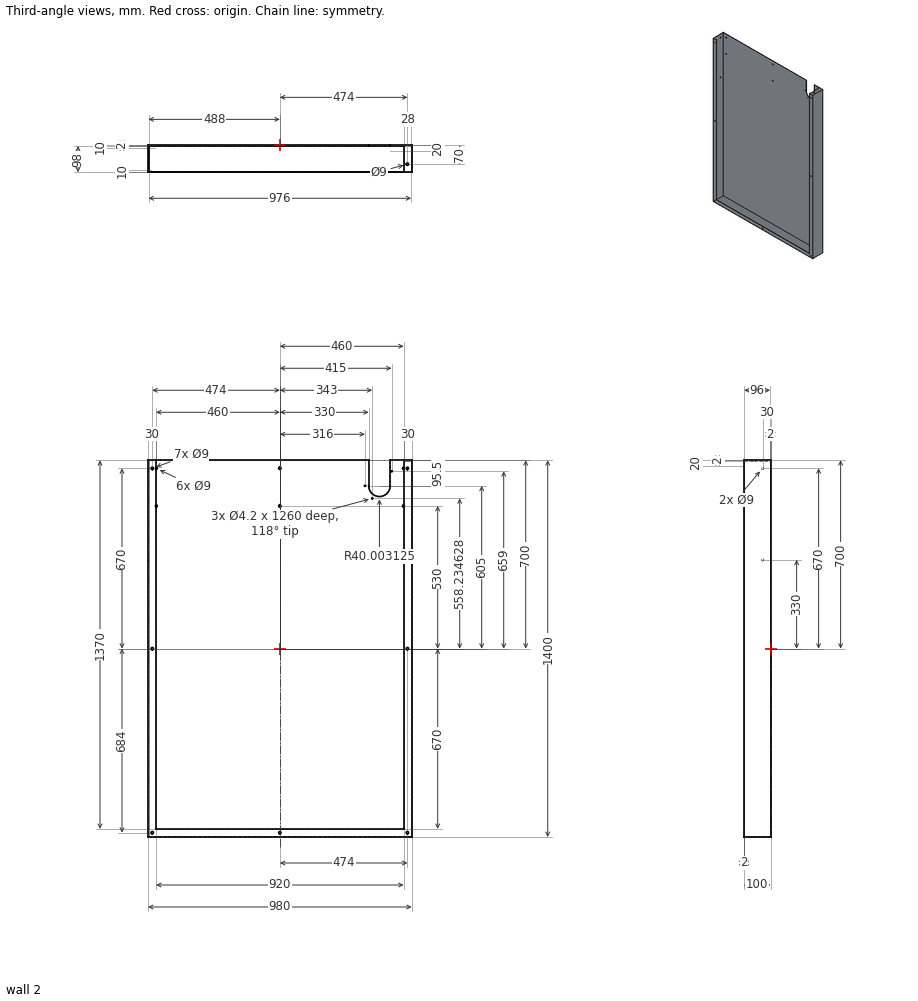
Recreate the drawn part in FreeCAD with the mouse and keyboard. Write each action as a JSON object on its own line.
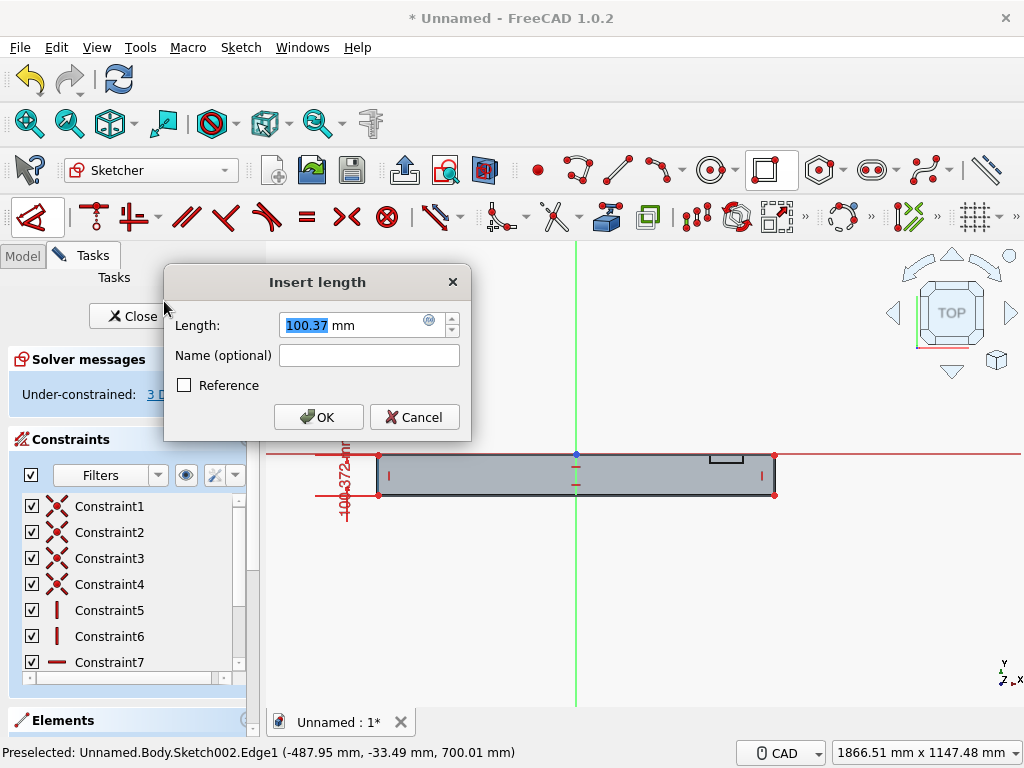
{"action": "type", "text": "98"}
{"action": "key", "text": "Return"}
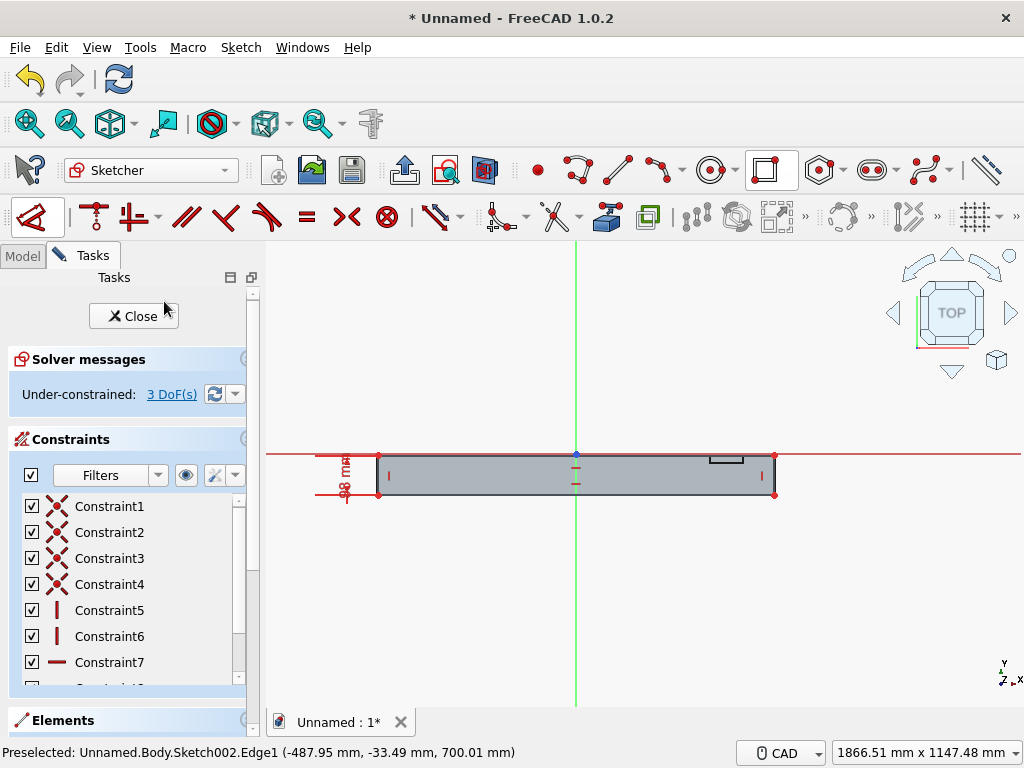
{"action": "scroll", "coordinate": [378, 456], "scroll_direction": "up", "scroll_amount": 20}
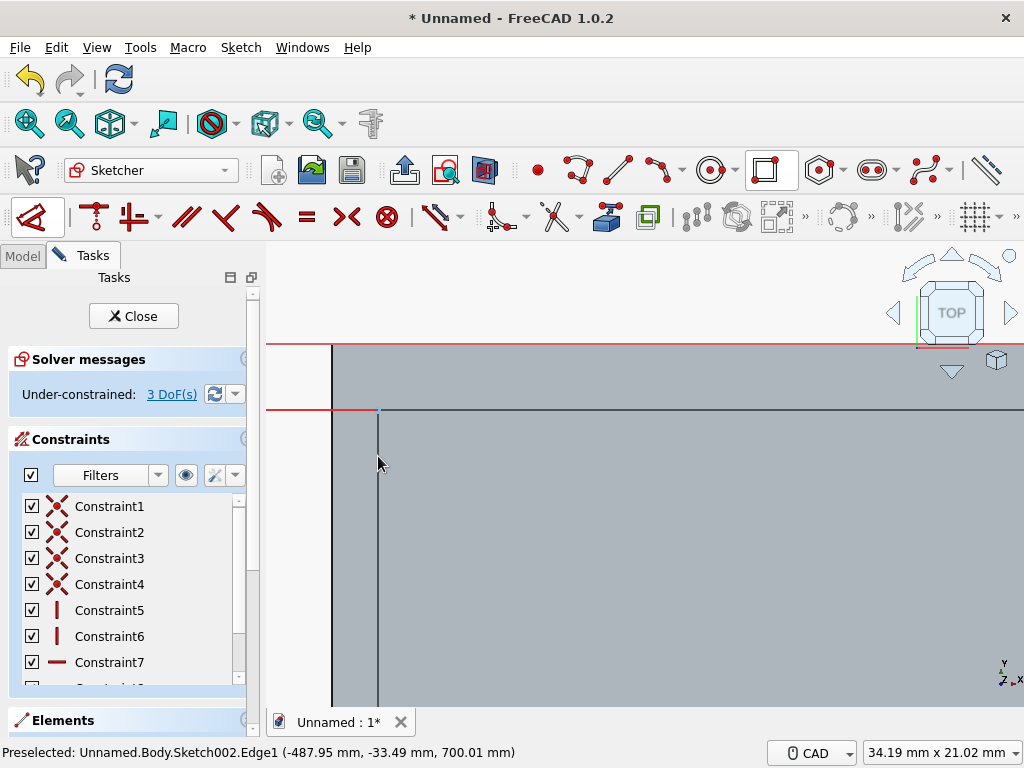
{"action": "left_click", "coordinate": [378, 410]}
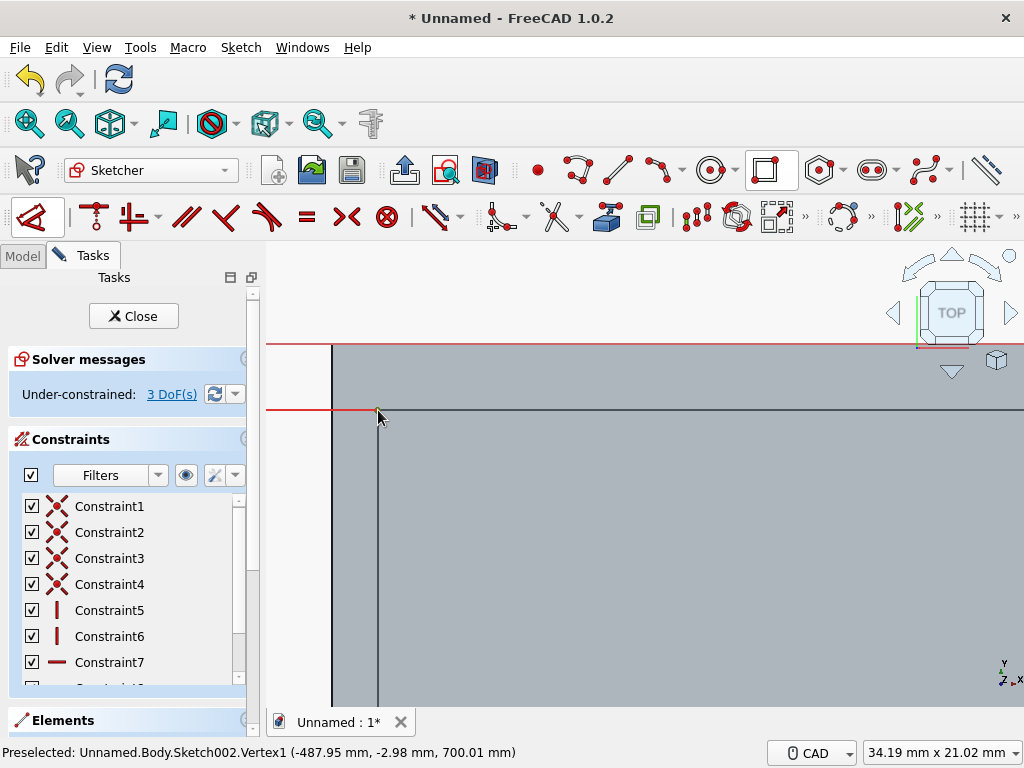
{"action": "key", "text": "i"}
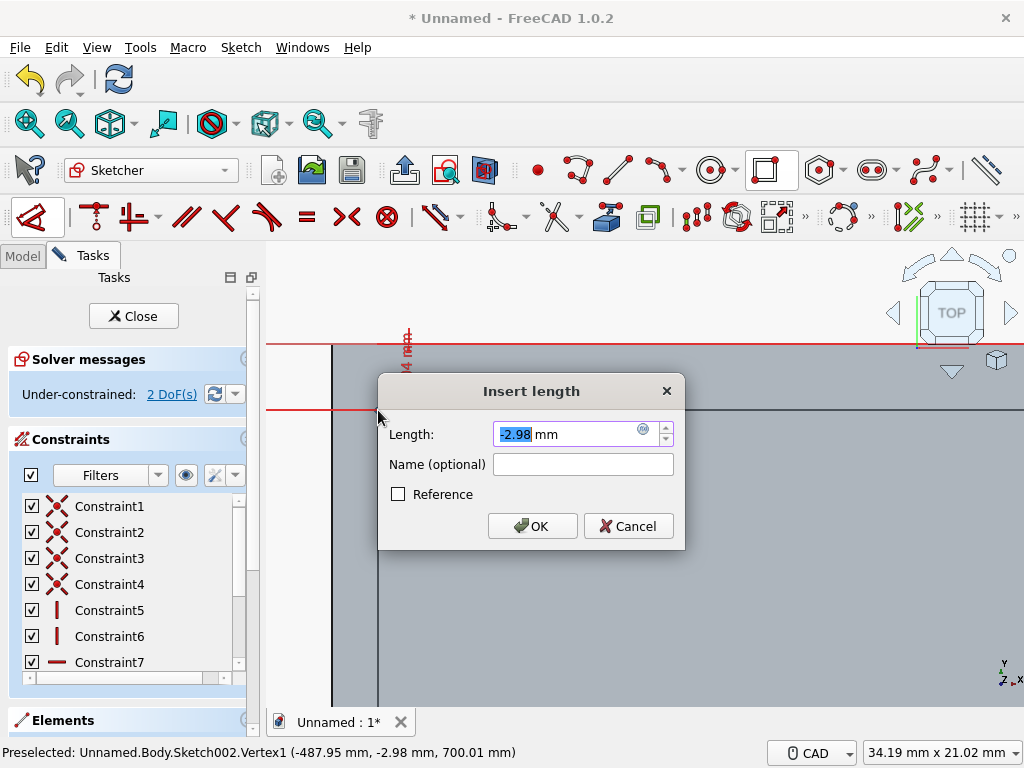
{"action": "type", "text": "-2"}
{"action": "key", "text": "Return"}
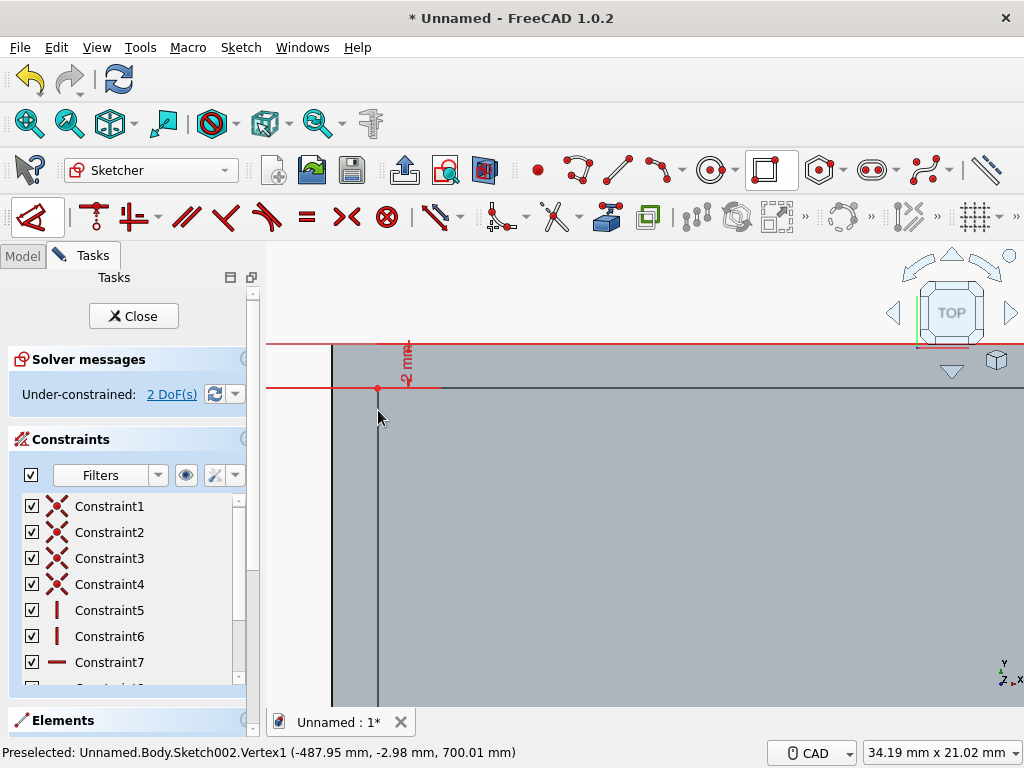
{"action": "scroll", "coordinate": [576, 474], "scroll_direction": "down", "scroll_amount": 15}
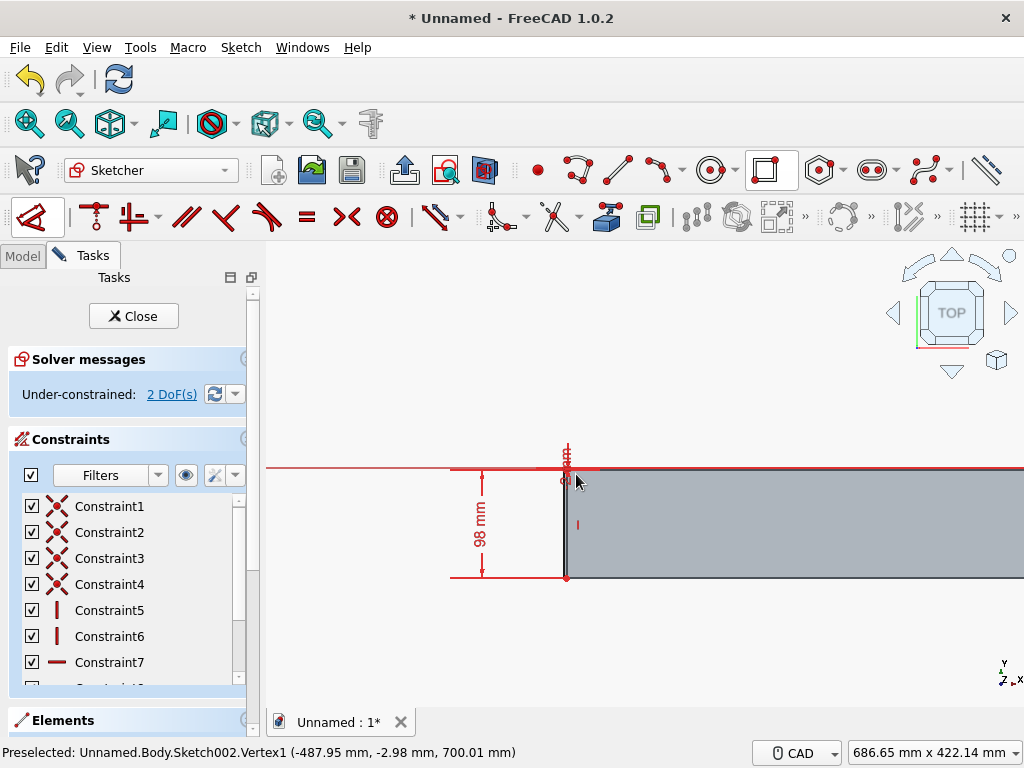
{"action": "scroll", "coordinate": [294, 445], "scroll_direction": "down", "scroll_amount": 5}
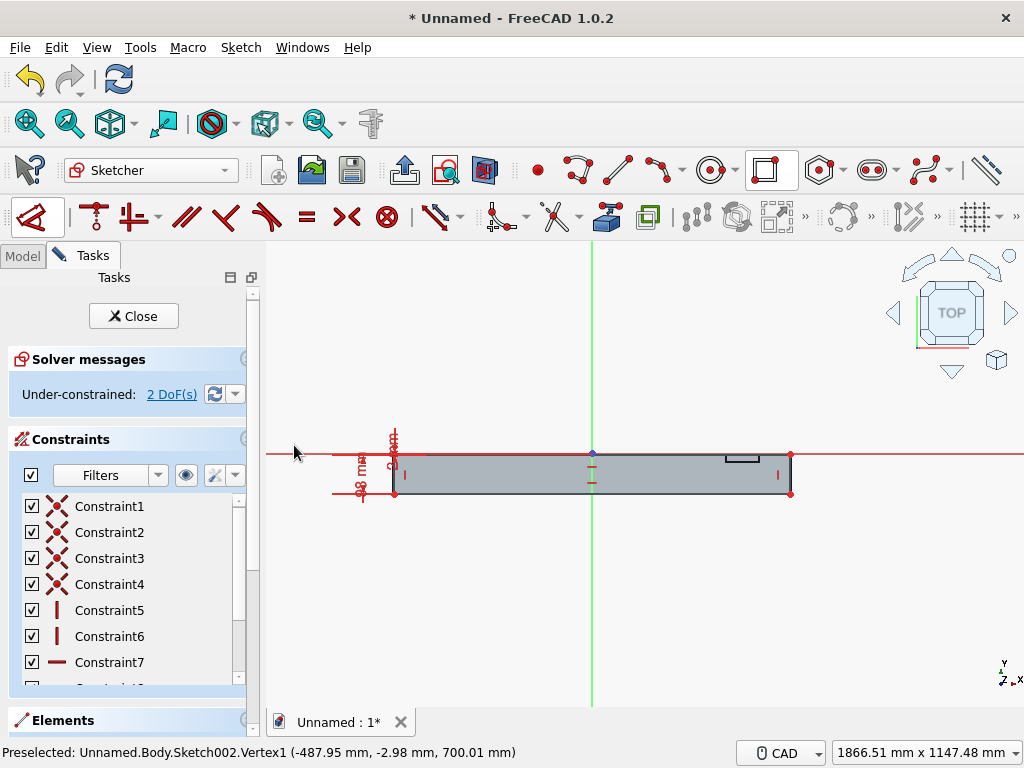
{"action": "left_click", "coordinate": [513, 494]}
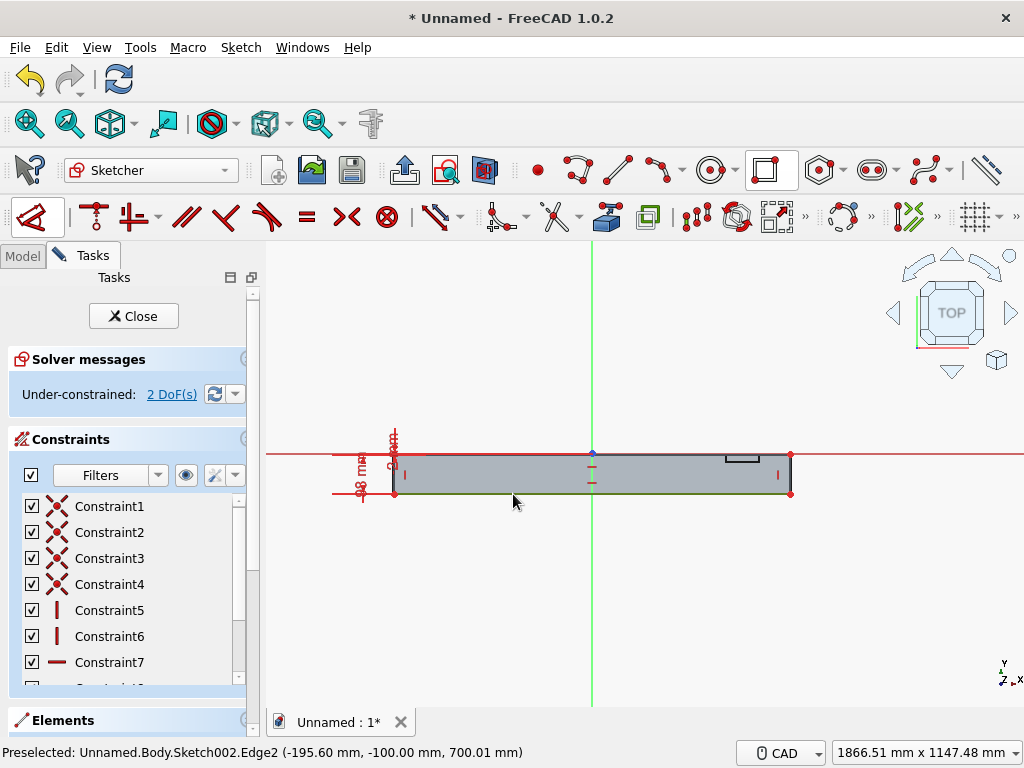
{"action": "left_click", "coordinate": [58, 218]}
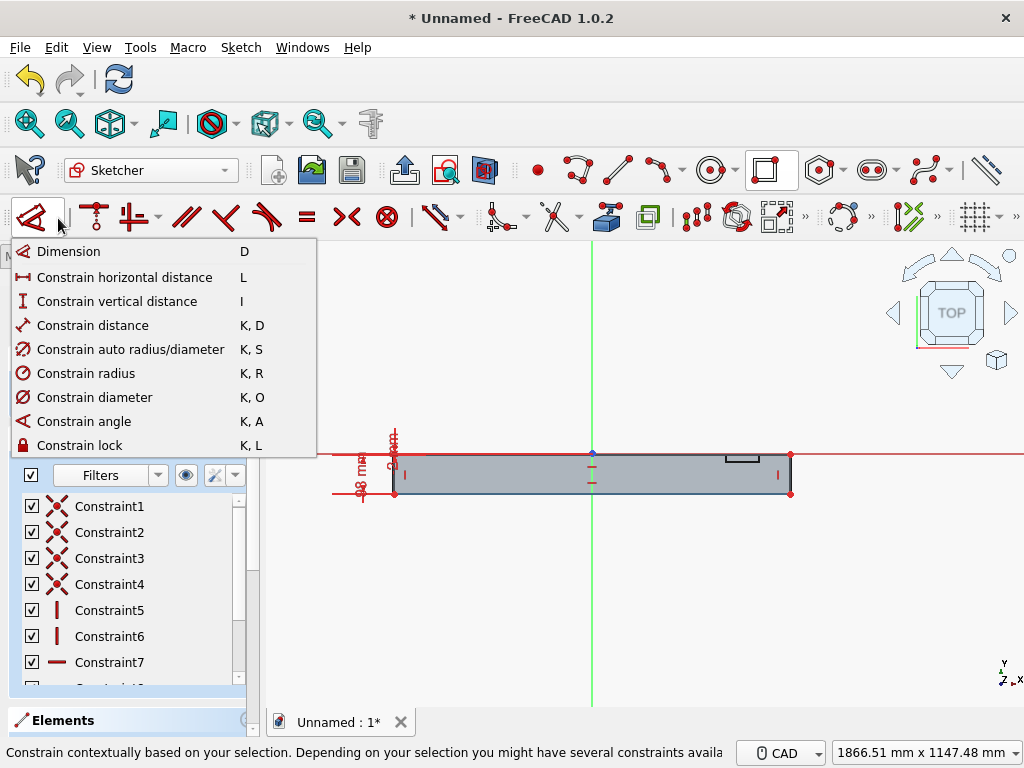
{"action": "left_click", "coordinate": [164, 277]}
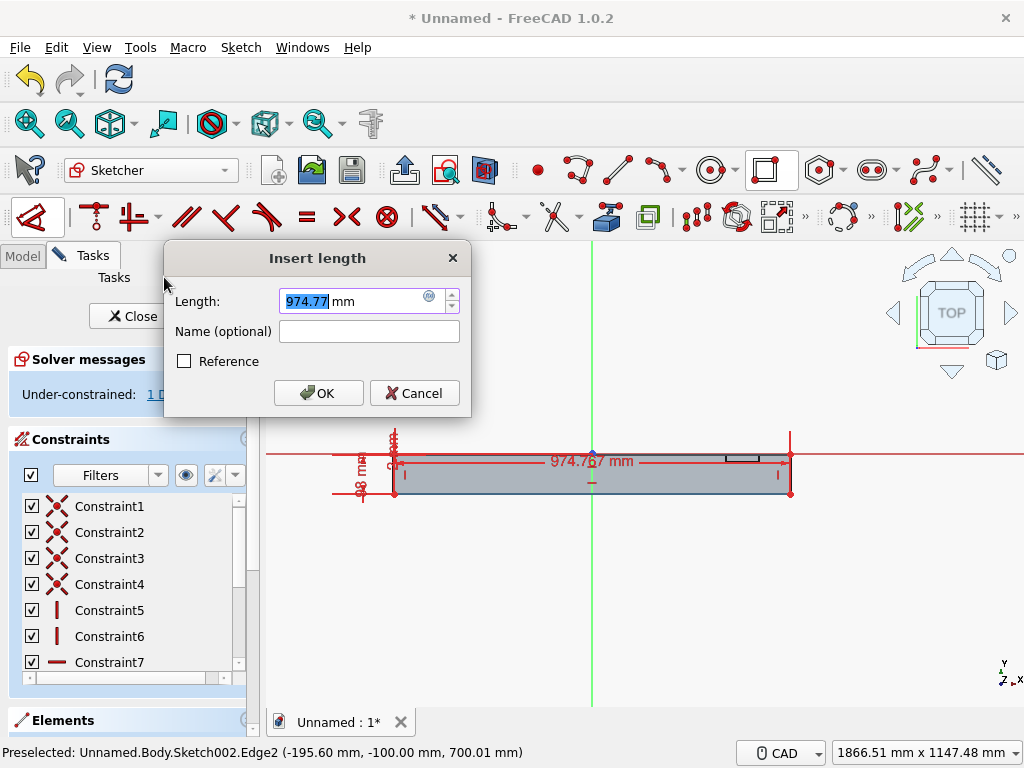
{"action": "type", "text": "976"}
{"action": "key", "text": "Return"}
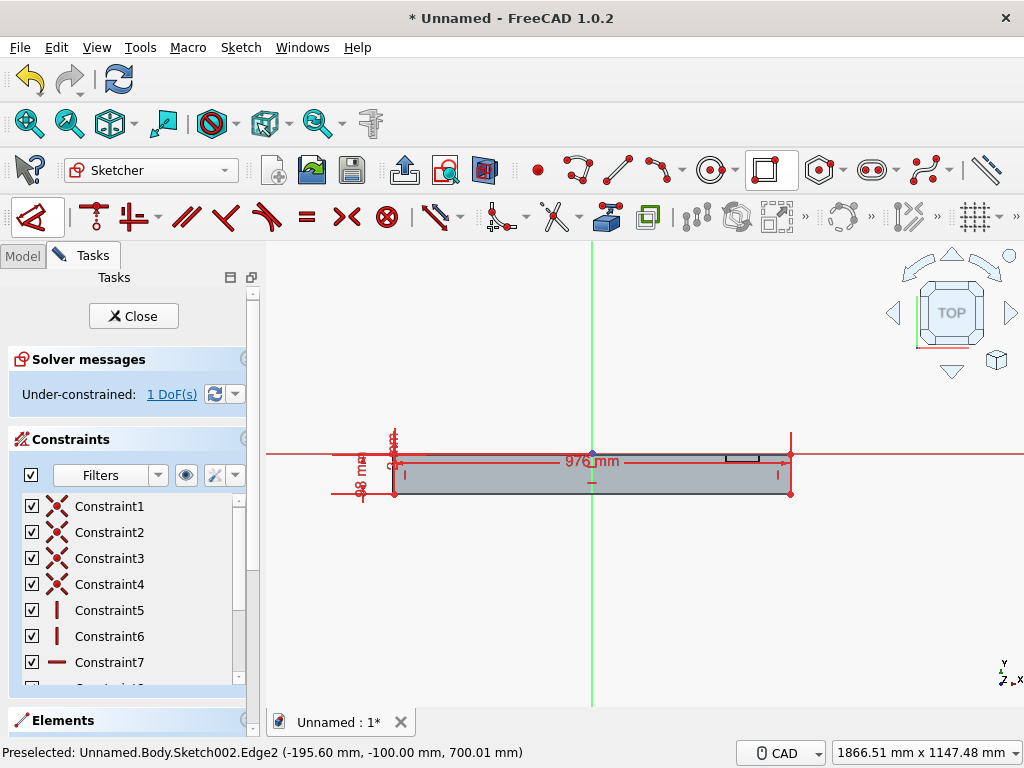
{"action": "left_click", "coordinate": [394, 455]}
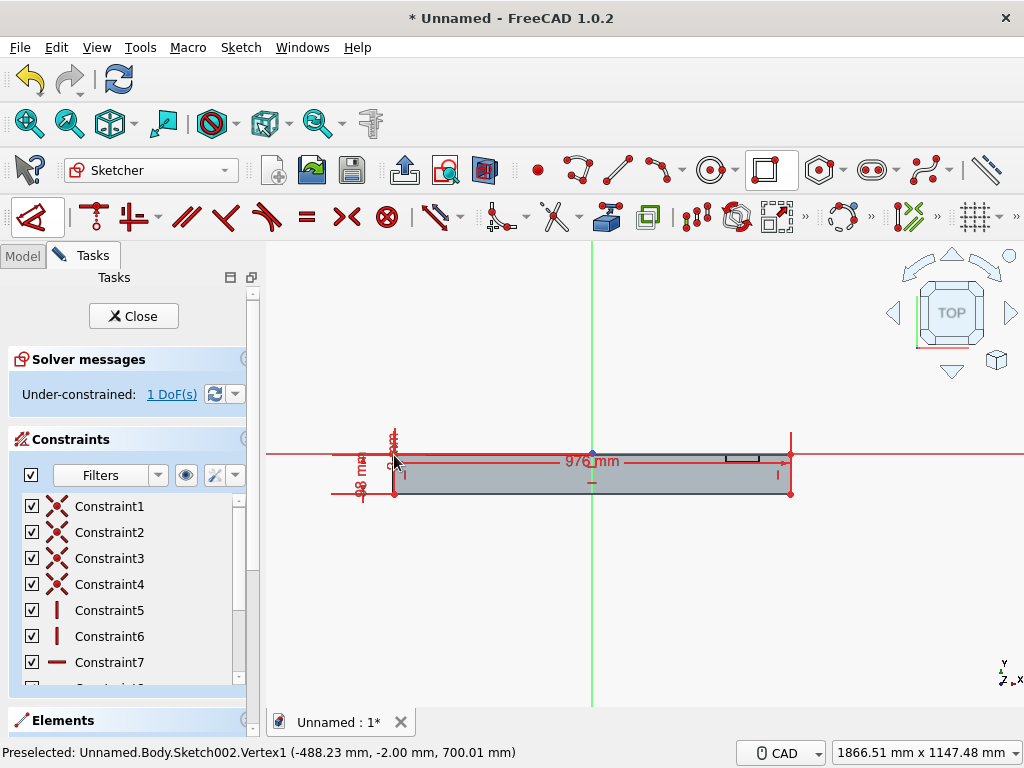
{"action": "left_click", "coordinate": [58, 218]}